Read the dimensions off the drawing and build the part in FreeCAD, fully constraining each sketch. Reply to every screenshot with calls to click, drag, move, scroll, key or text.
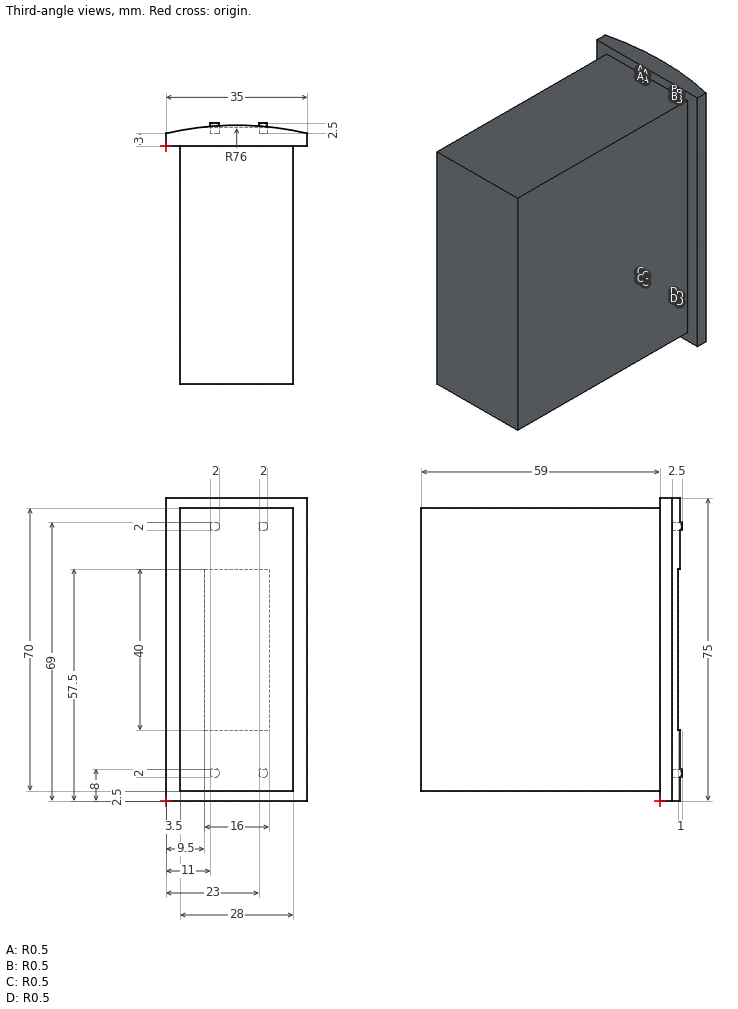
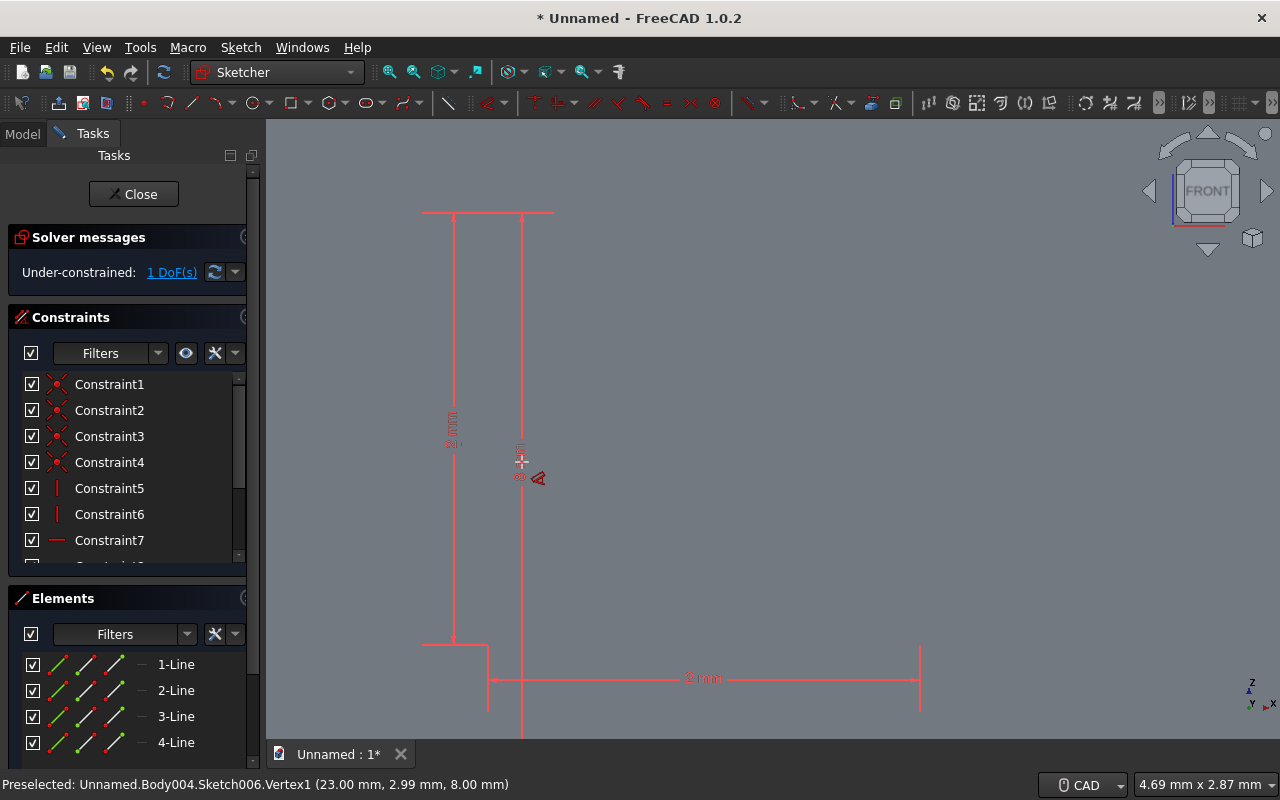
click(488, 213)
click(391, 179)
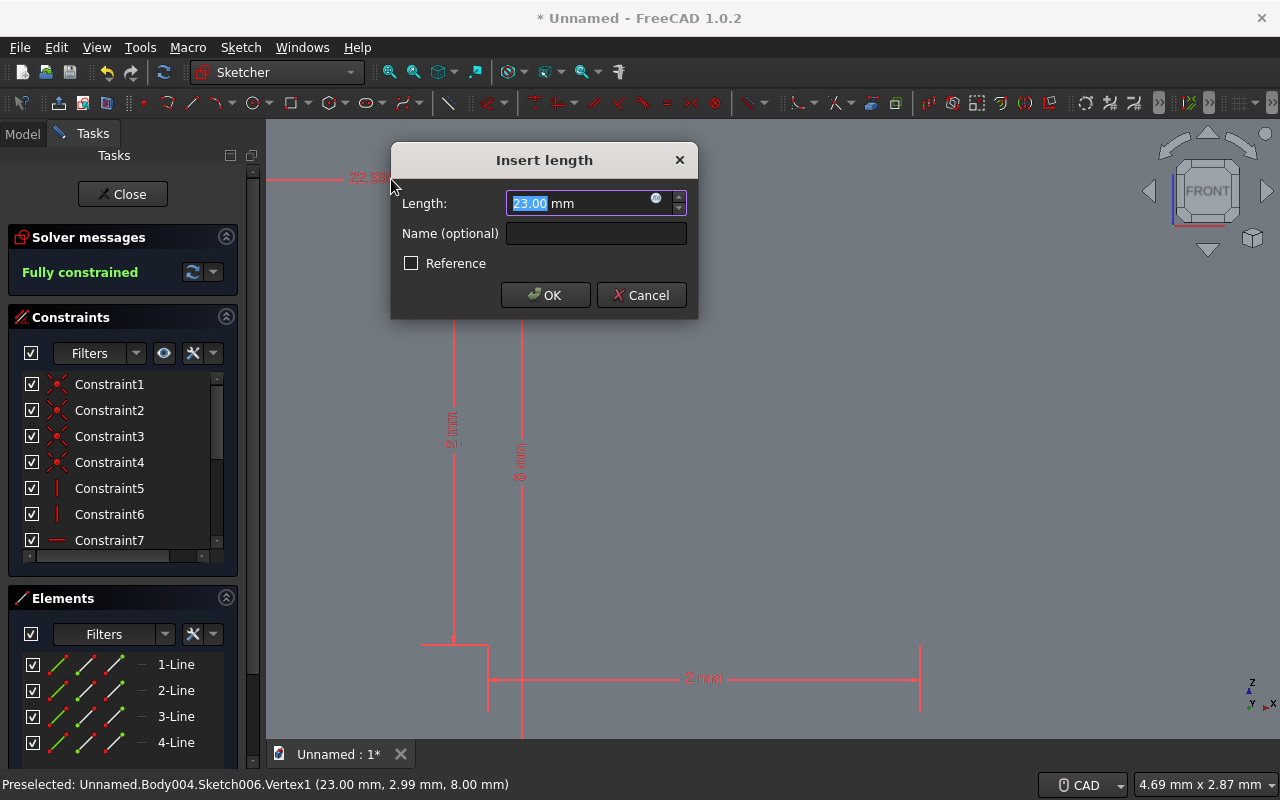
text(23)
key(Return)
key(Escape)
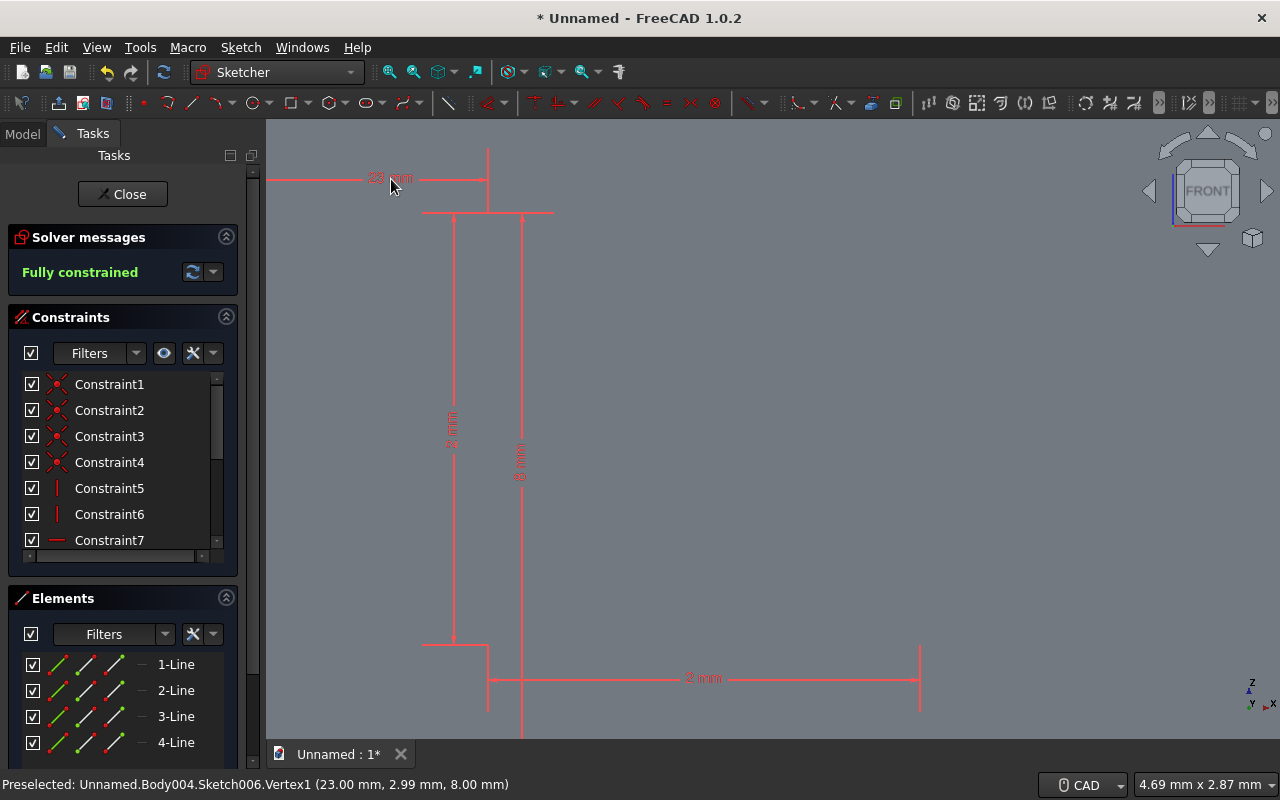
click(123, 194)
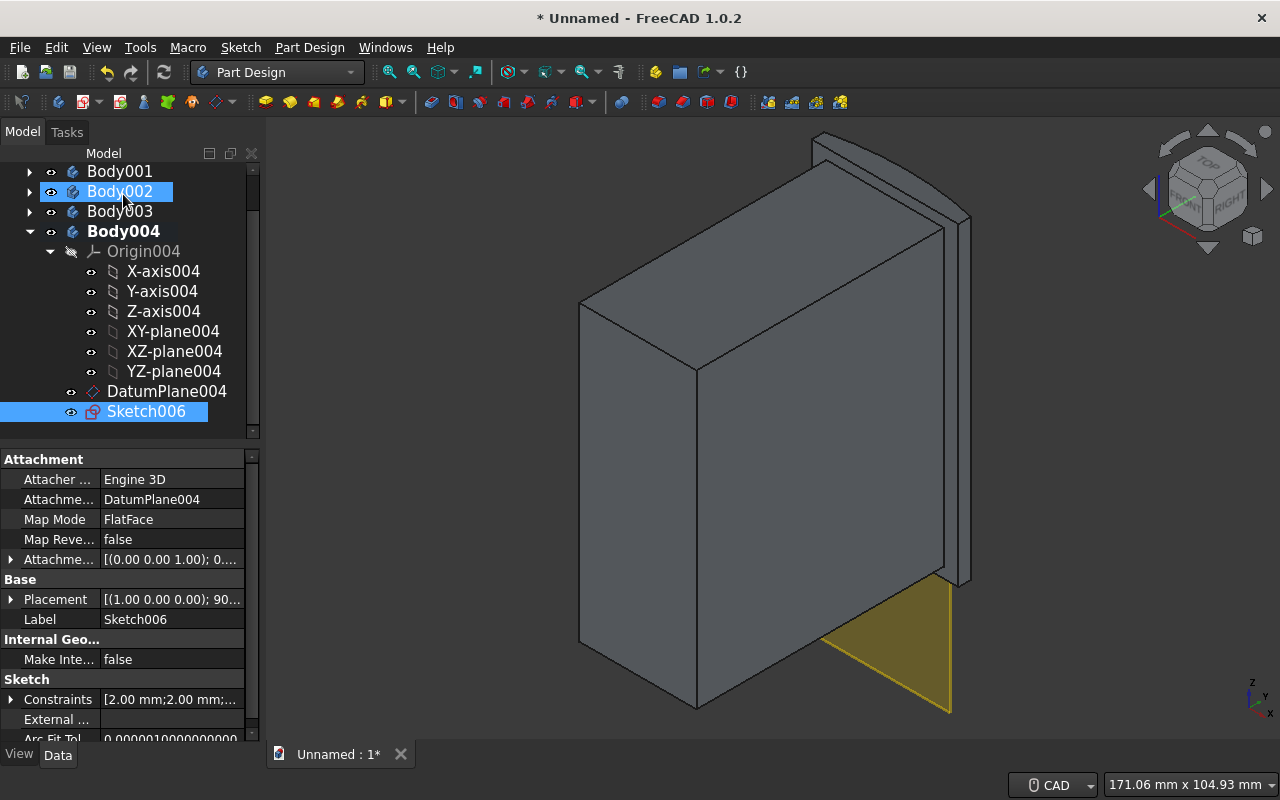
click(266, 102)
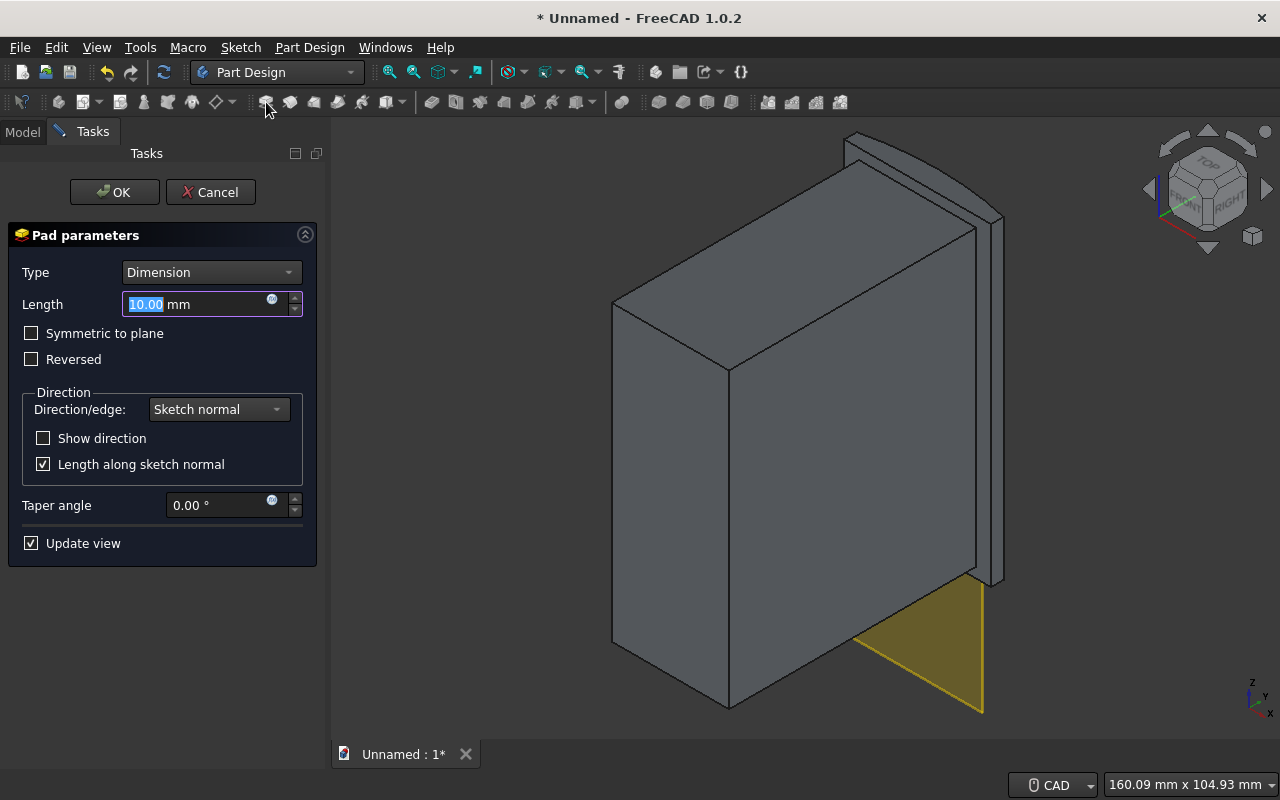
text(2.5)
key(Tab)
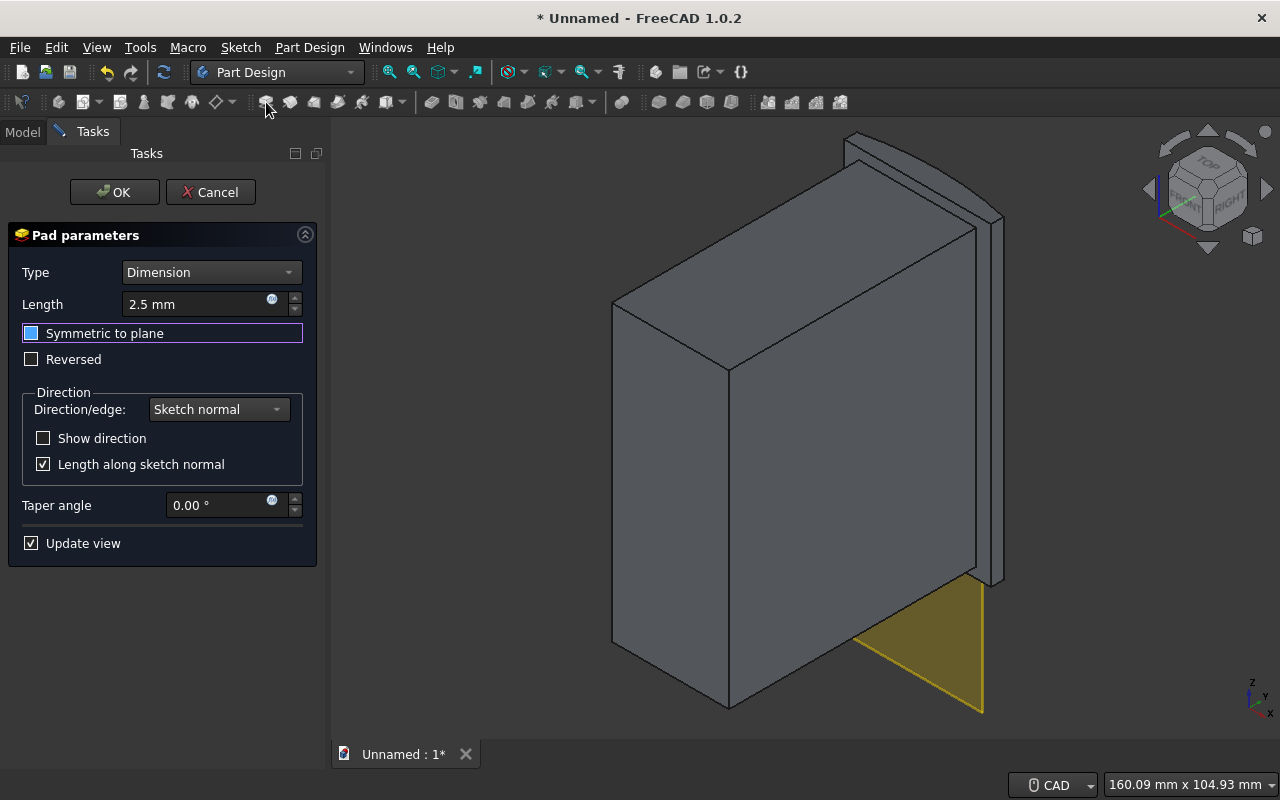
click(30, 359)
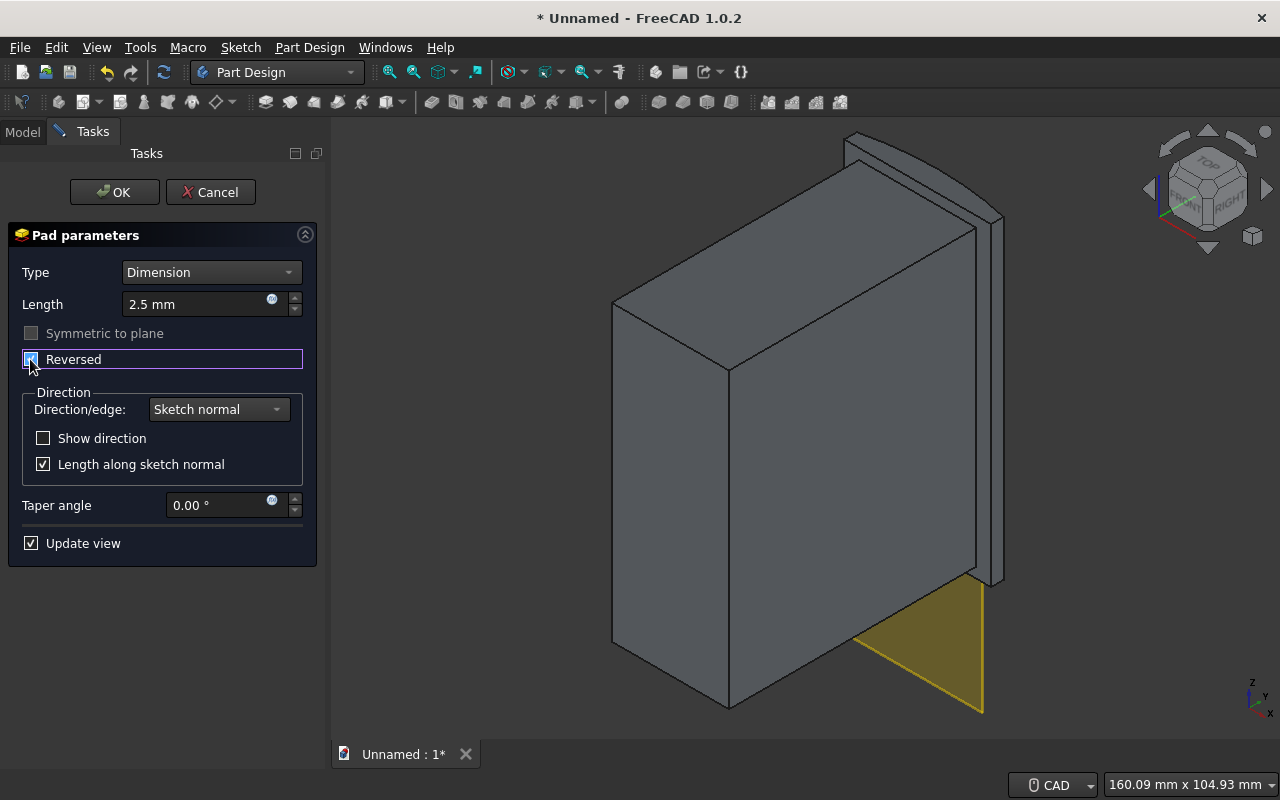
click(115, 192)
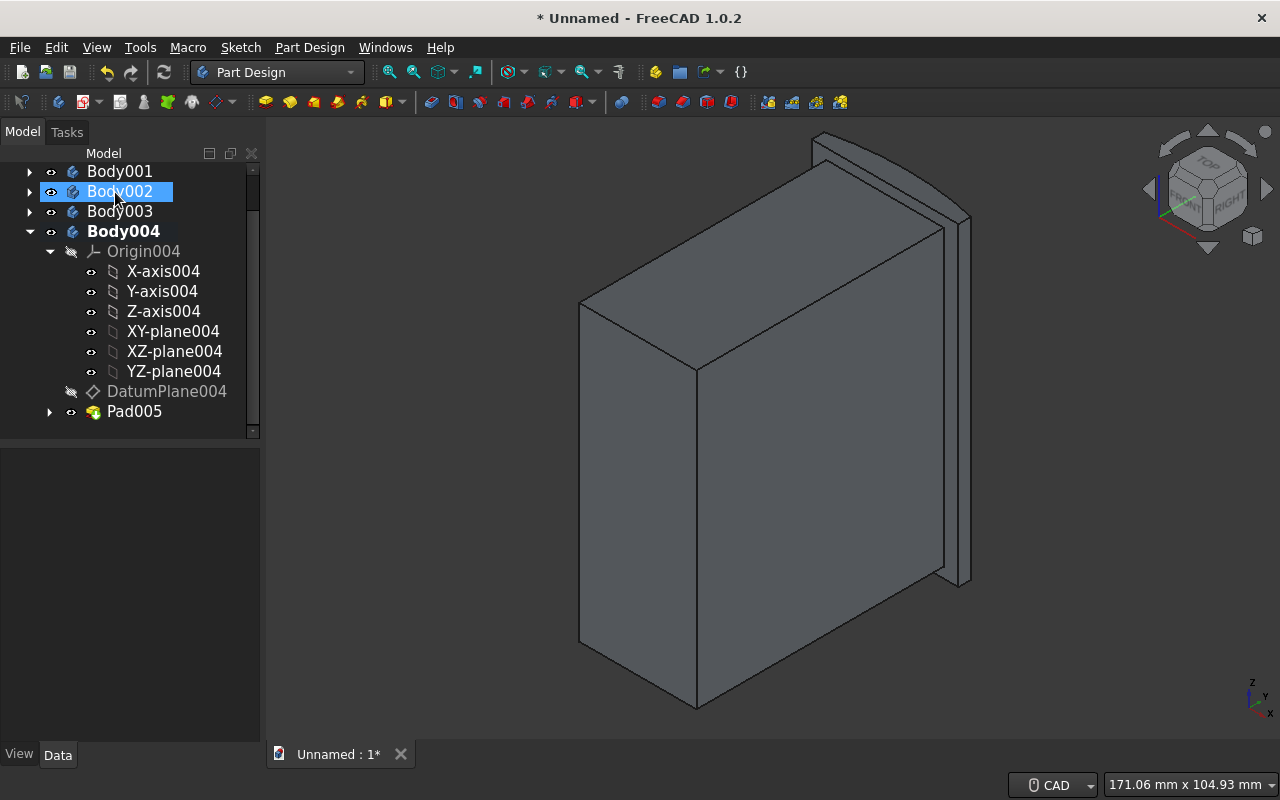
key(v)
key(f)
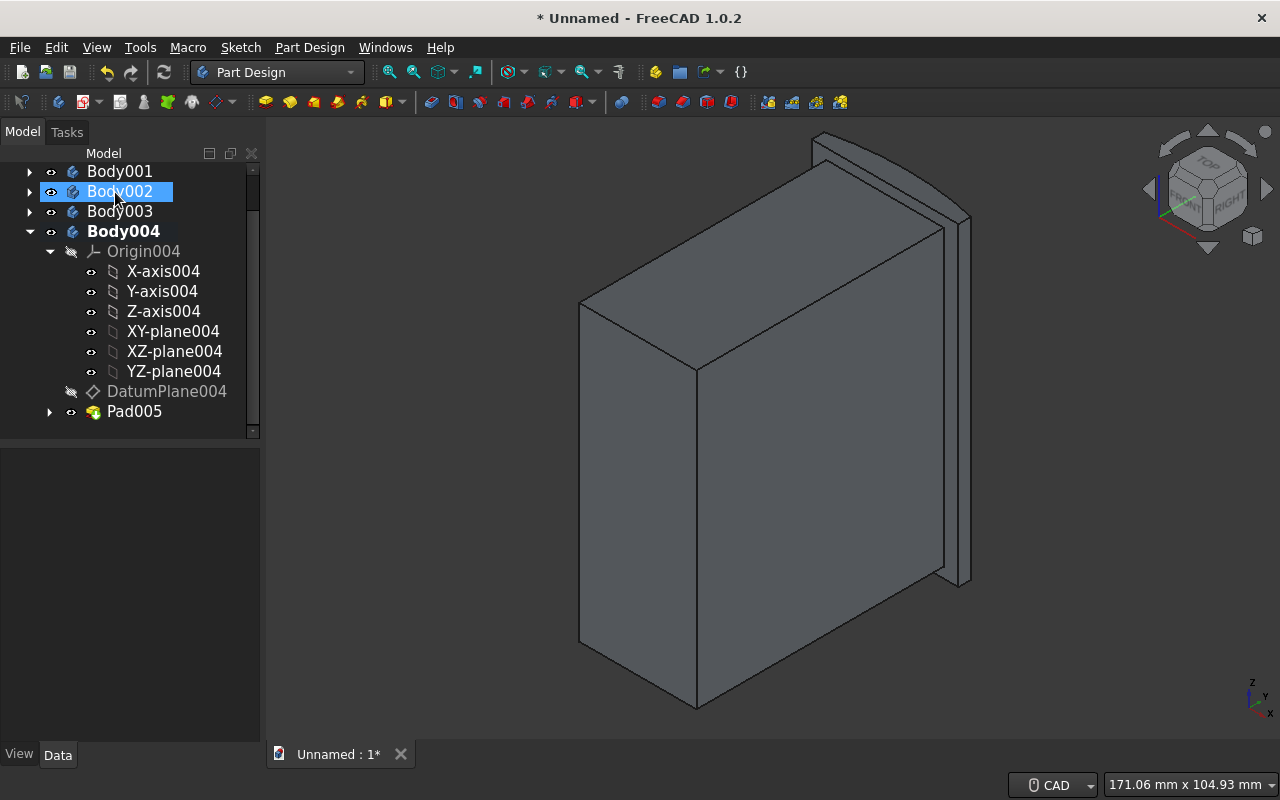
scroll(926, 508, up, 5)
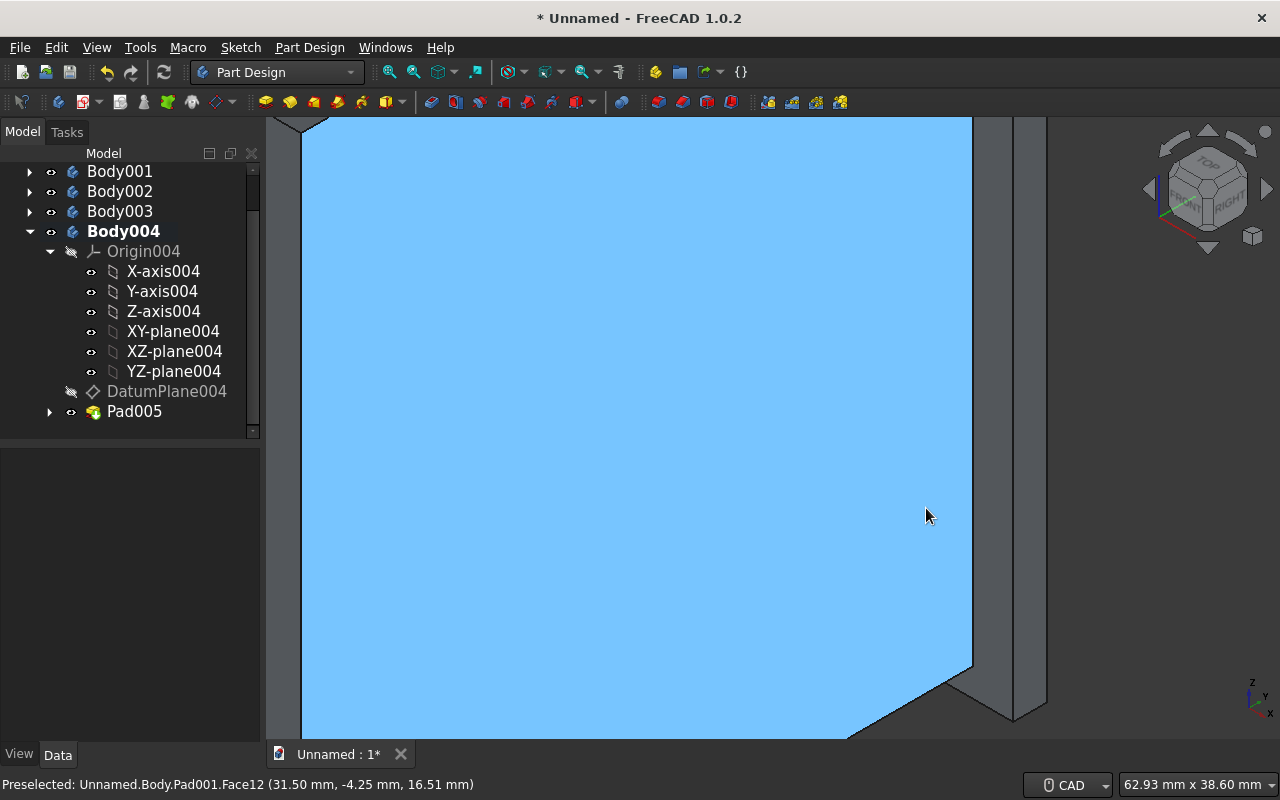
key(v)
key(f)